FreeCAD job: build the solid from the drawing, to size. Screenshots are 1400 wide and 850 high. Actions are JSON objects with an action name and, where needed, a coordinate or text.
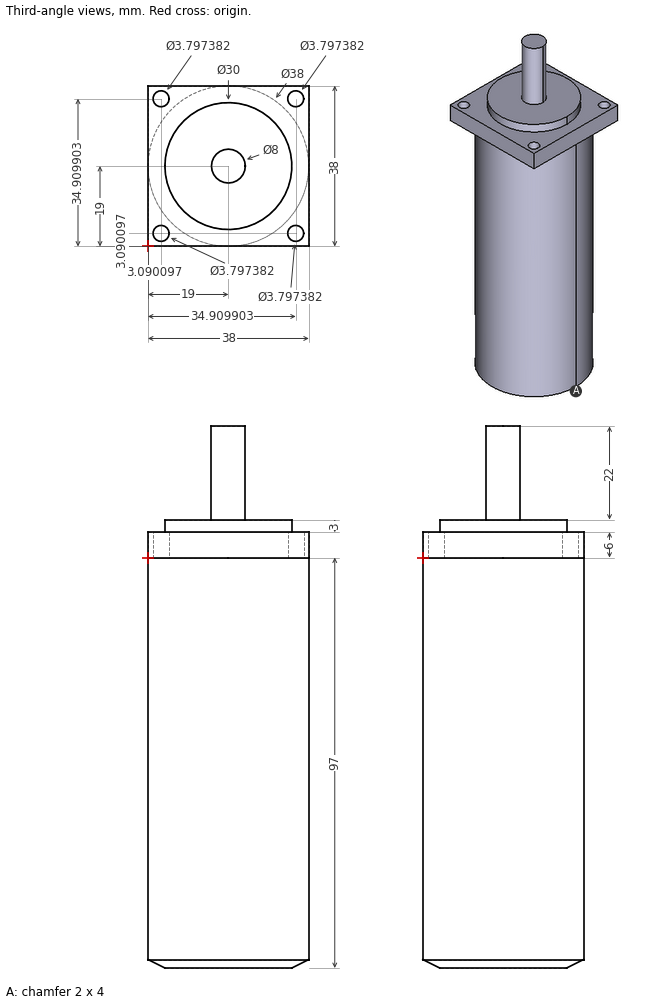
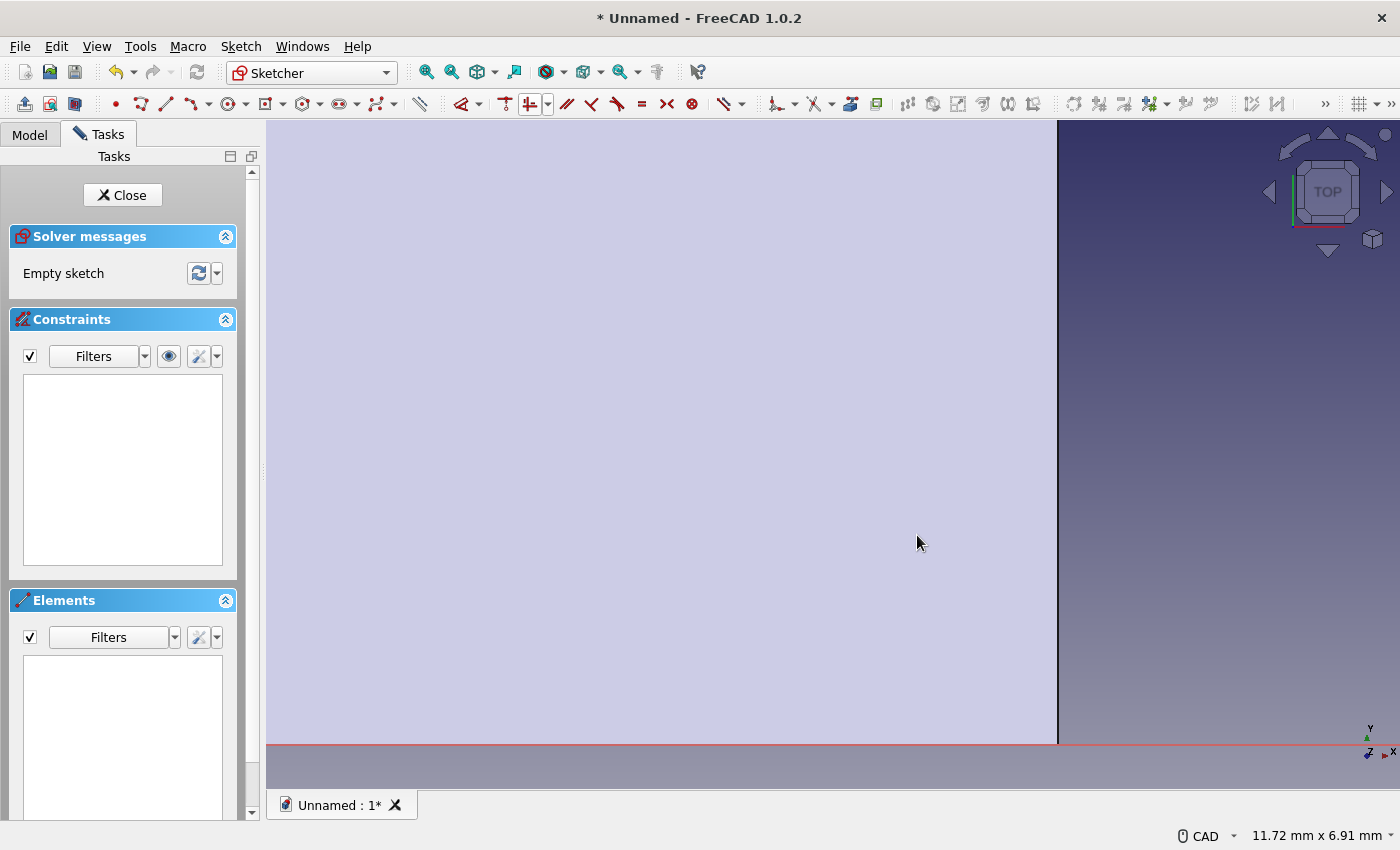
{"action": "key", "text": "g c"}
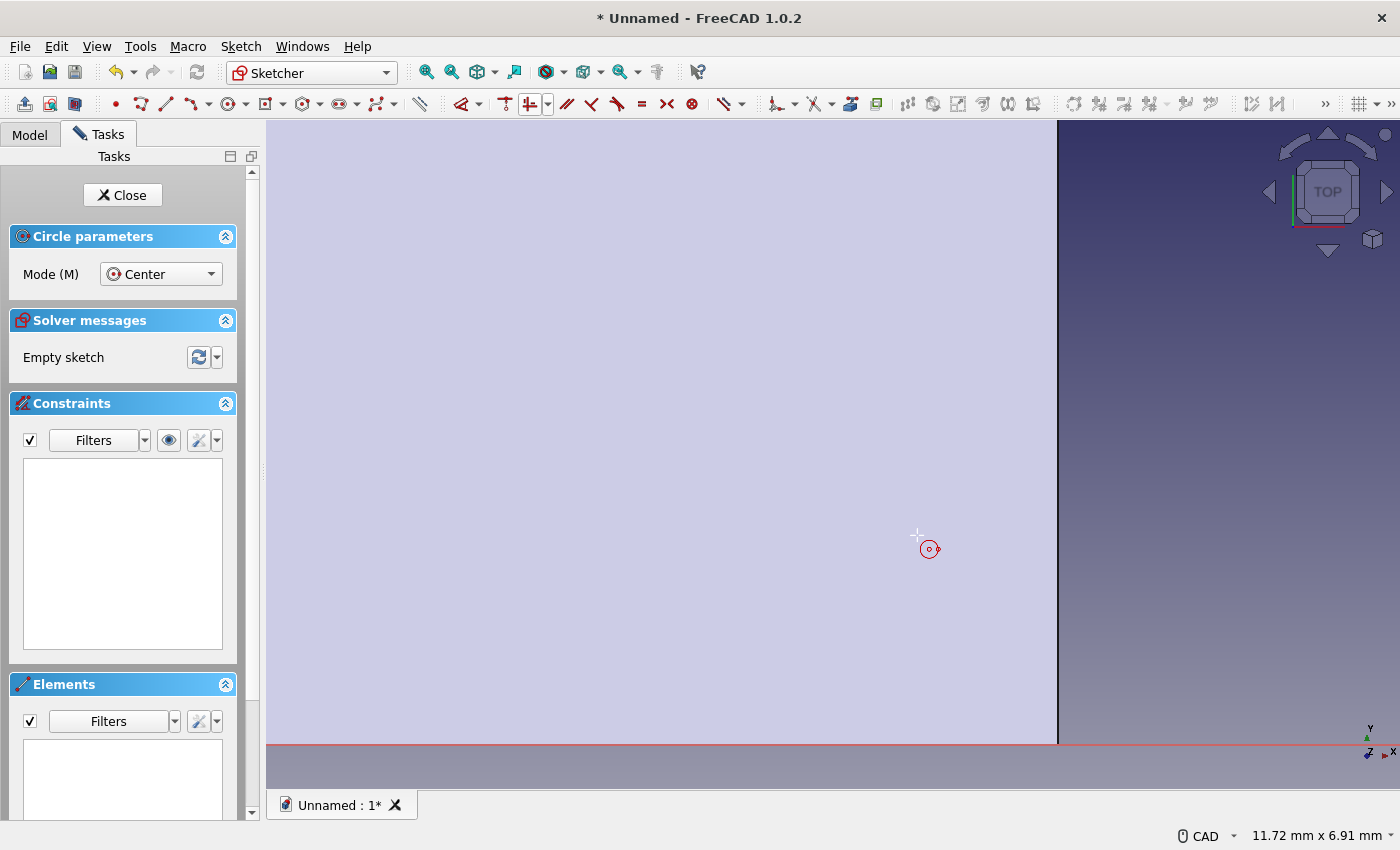
{"action": "left_click", "coordinate": [759, 446]}
{"action": "mouse_move", "coordinate": [889, 316]}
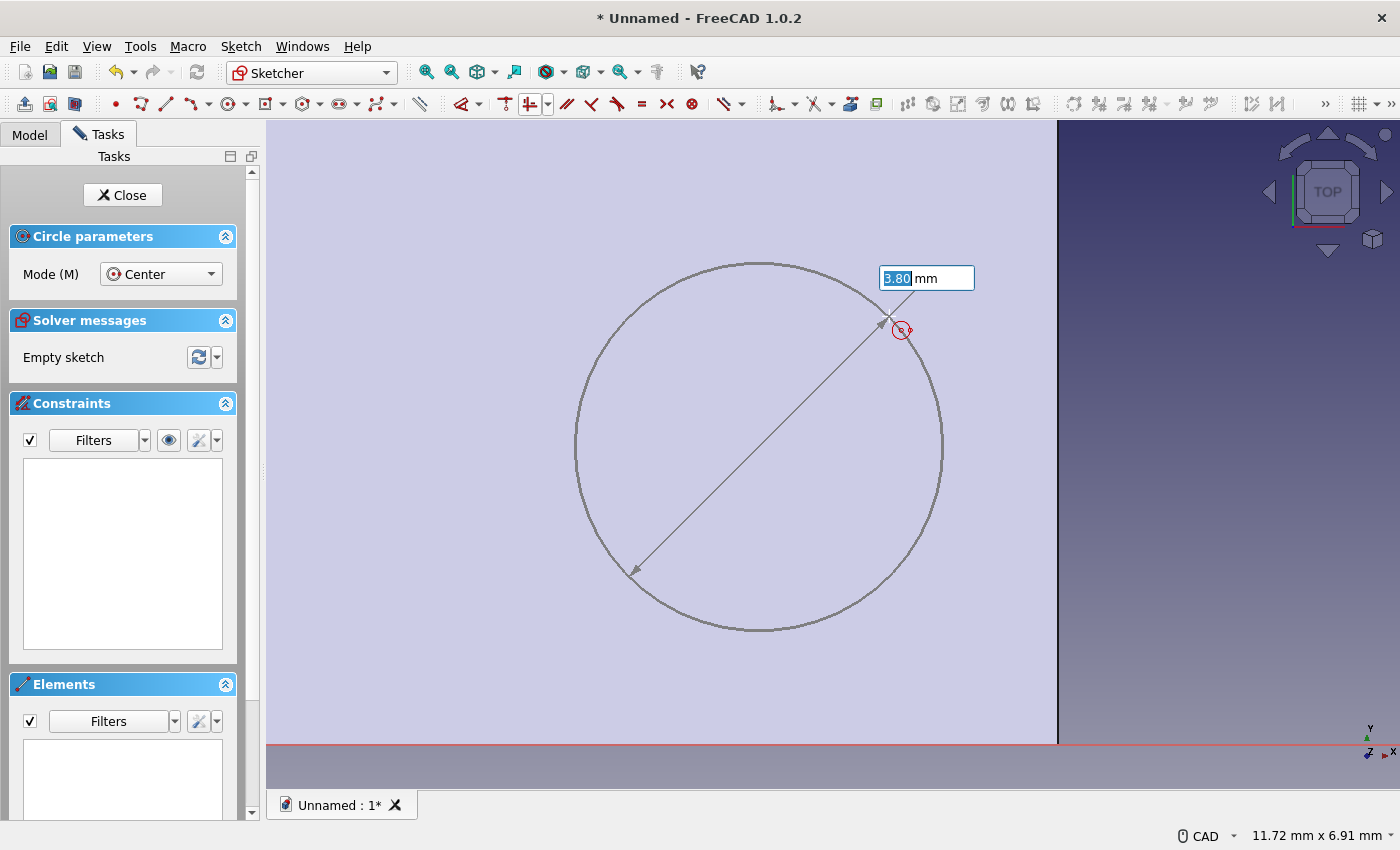
{"action": "type", "text": "3.797382"}
{"action": "key", "text": "Return"}
{"action": "key", "text": "Escape"}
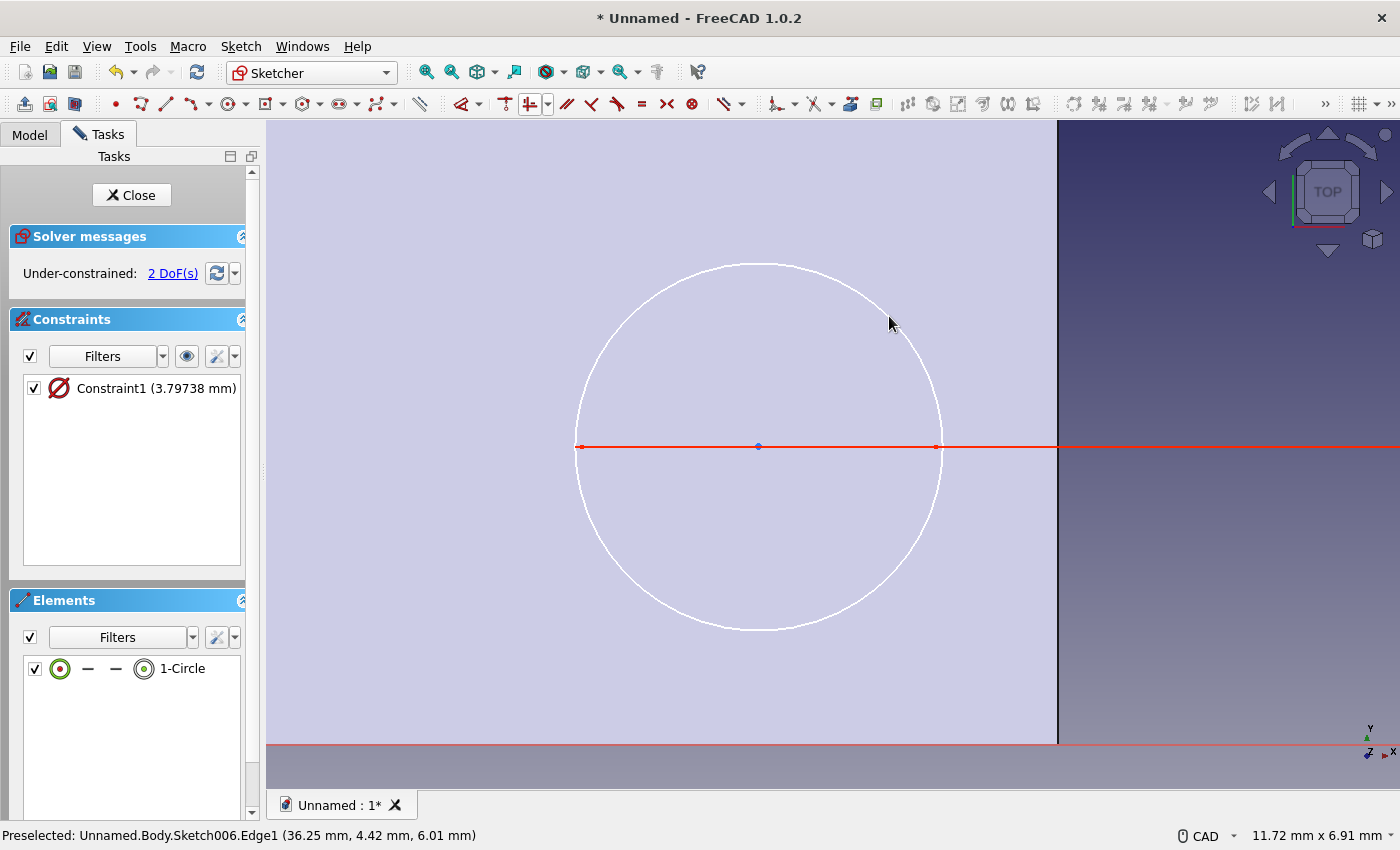
{"action": "key", "text": "d"}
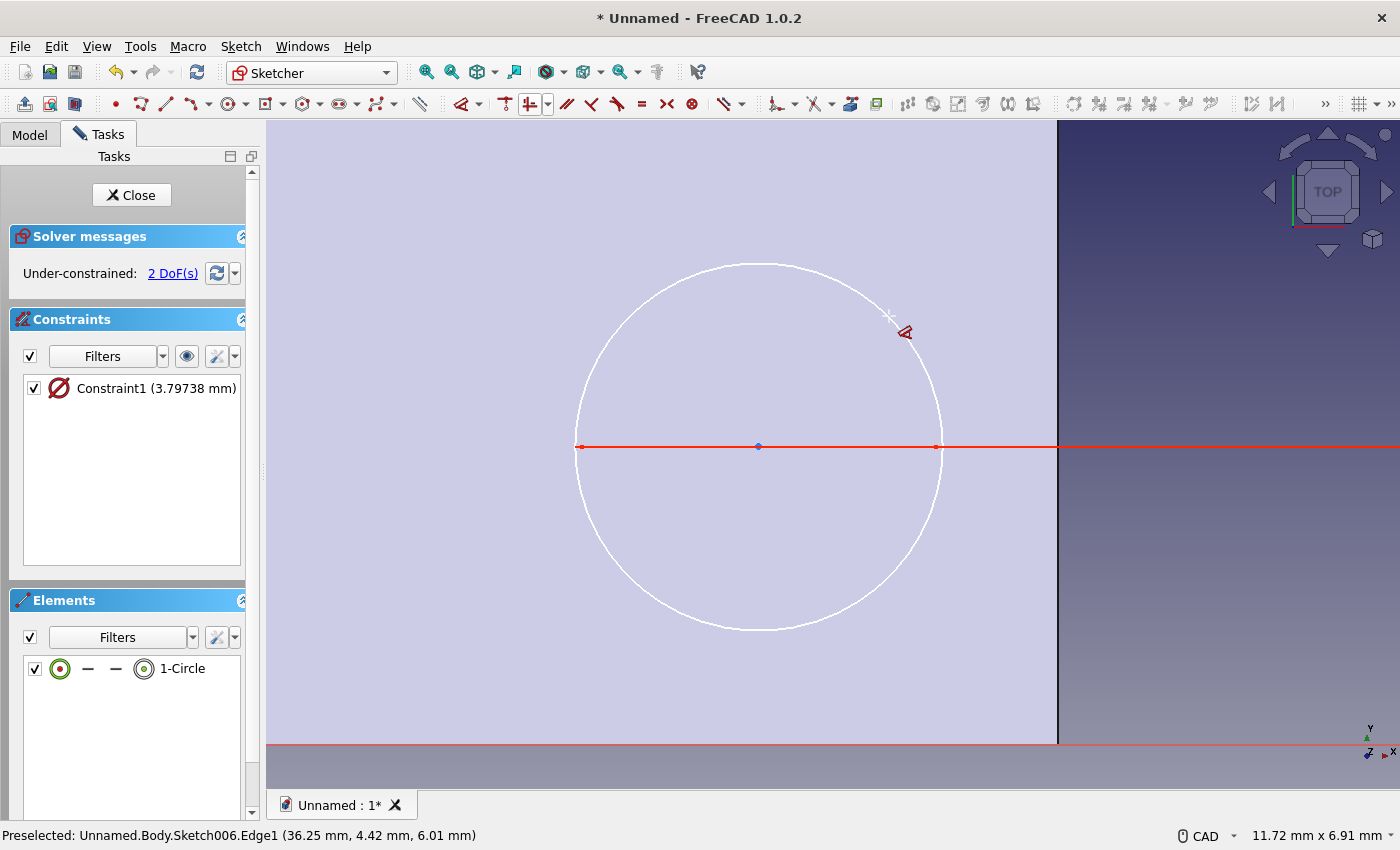
{"action": "left_click", "coordinate": [759, 447]}
{"action": "left_click", "coordinate": [793, 596]}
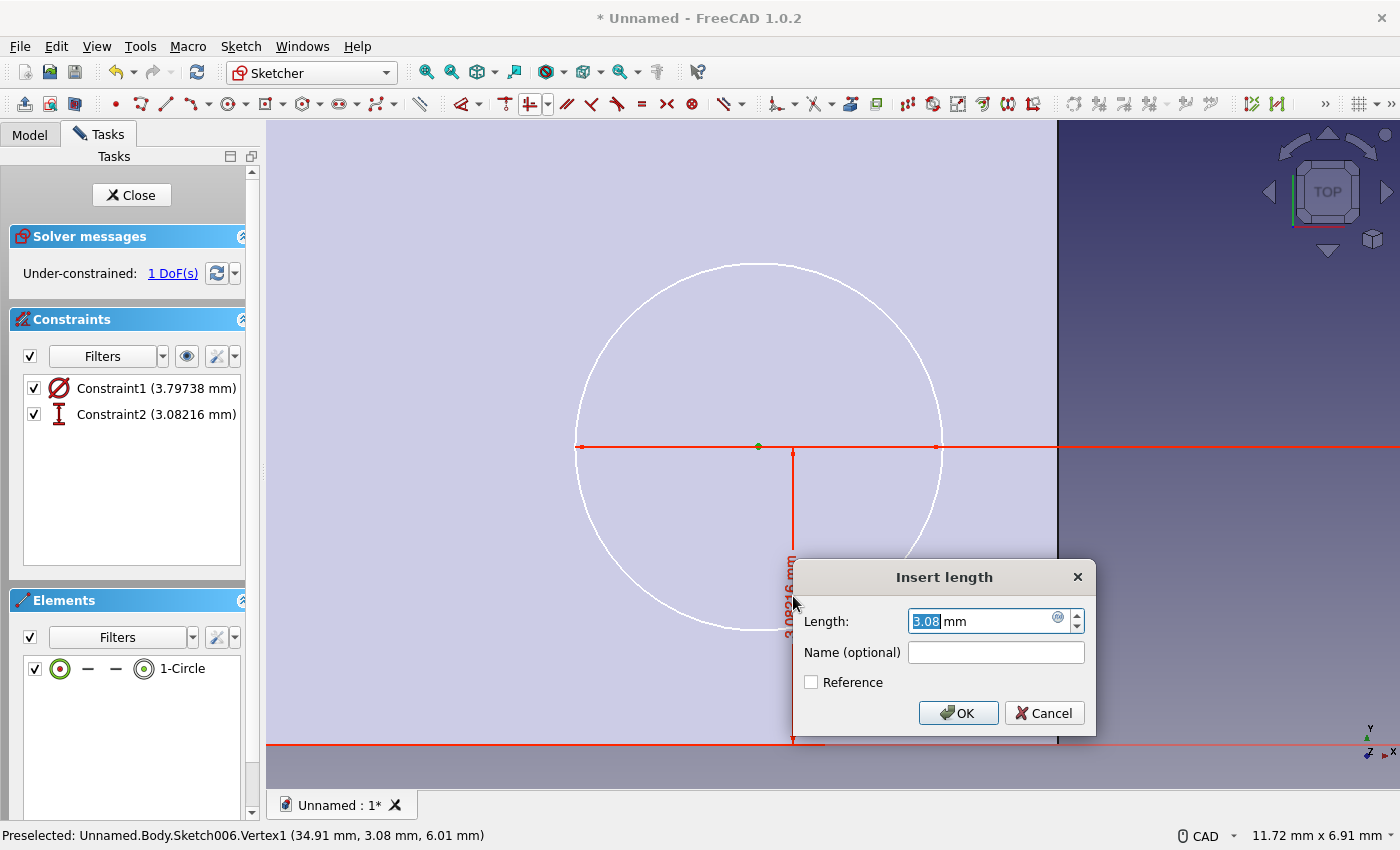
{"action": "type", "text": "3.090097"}
{"action": "key", "text": "Return"}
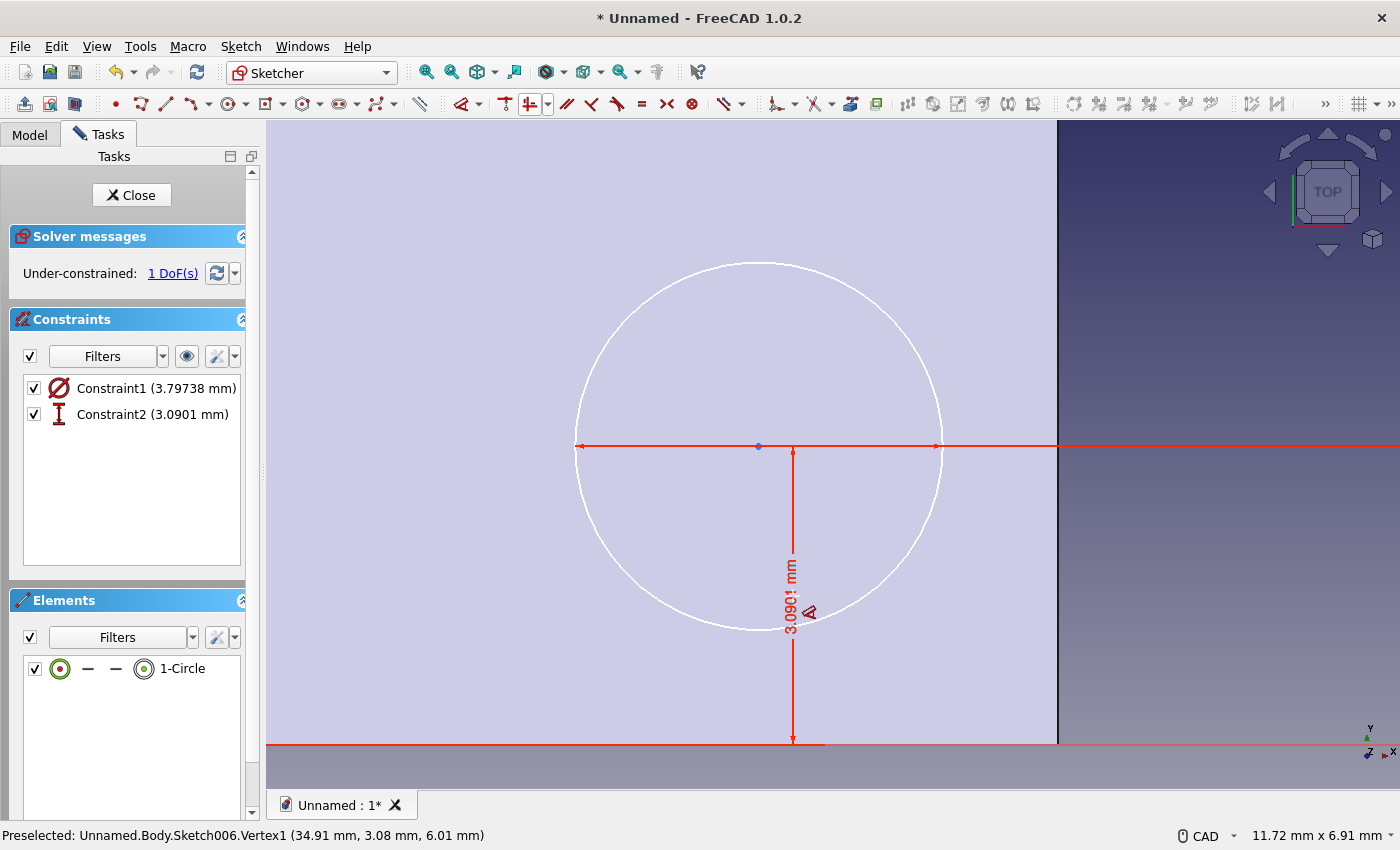
{"action": "left_click", "coordinate": [759, 446]}
{"action": "left_click", "coordinate": [526, 412]}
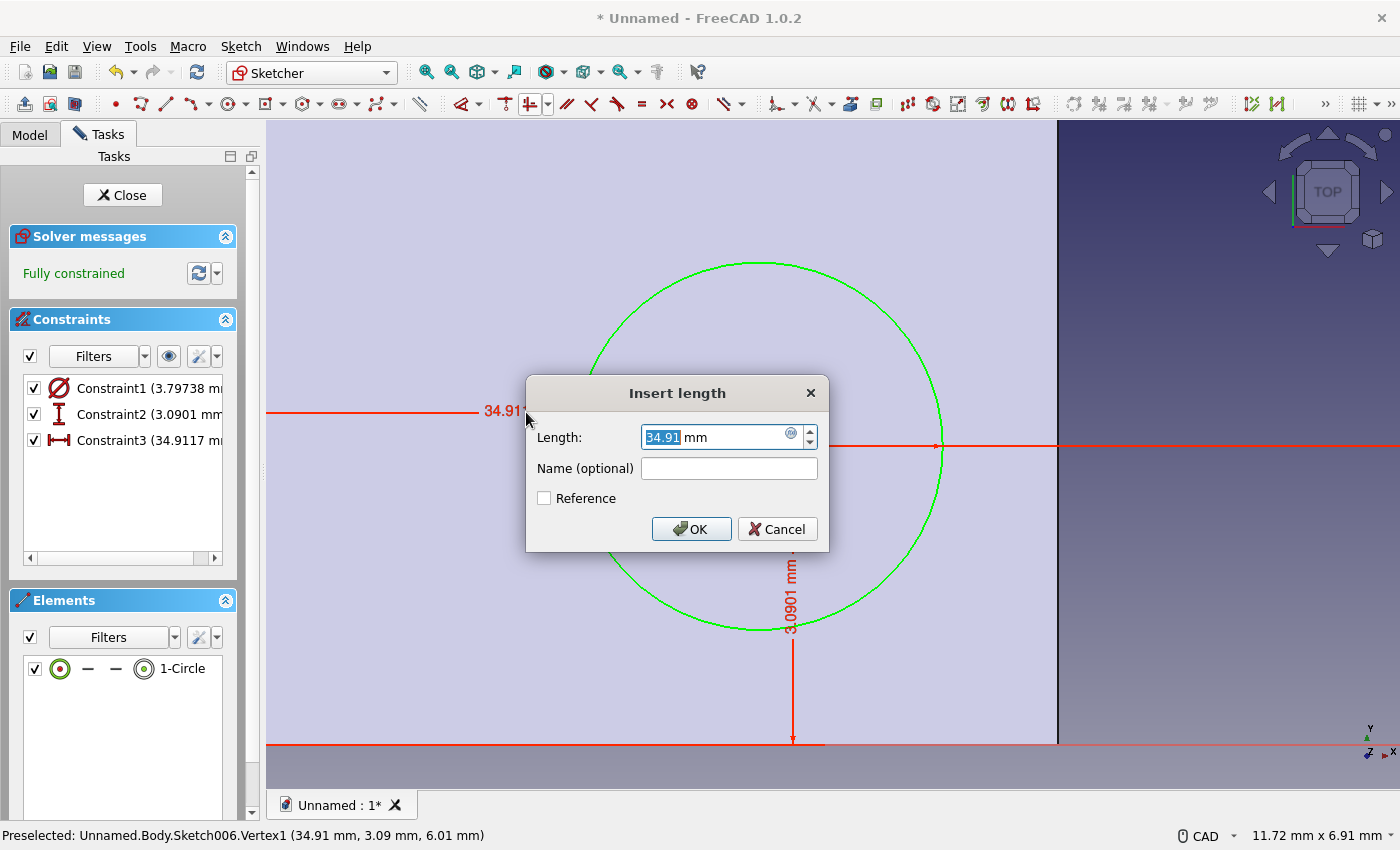
{"action": "type", "text": "34.909903"}
{"action": "key", "text": "Return"}
{"action": "key", "text": "Escape"}